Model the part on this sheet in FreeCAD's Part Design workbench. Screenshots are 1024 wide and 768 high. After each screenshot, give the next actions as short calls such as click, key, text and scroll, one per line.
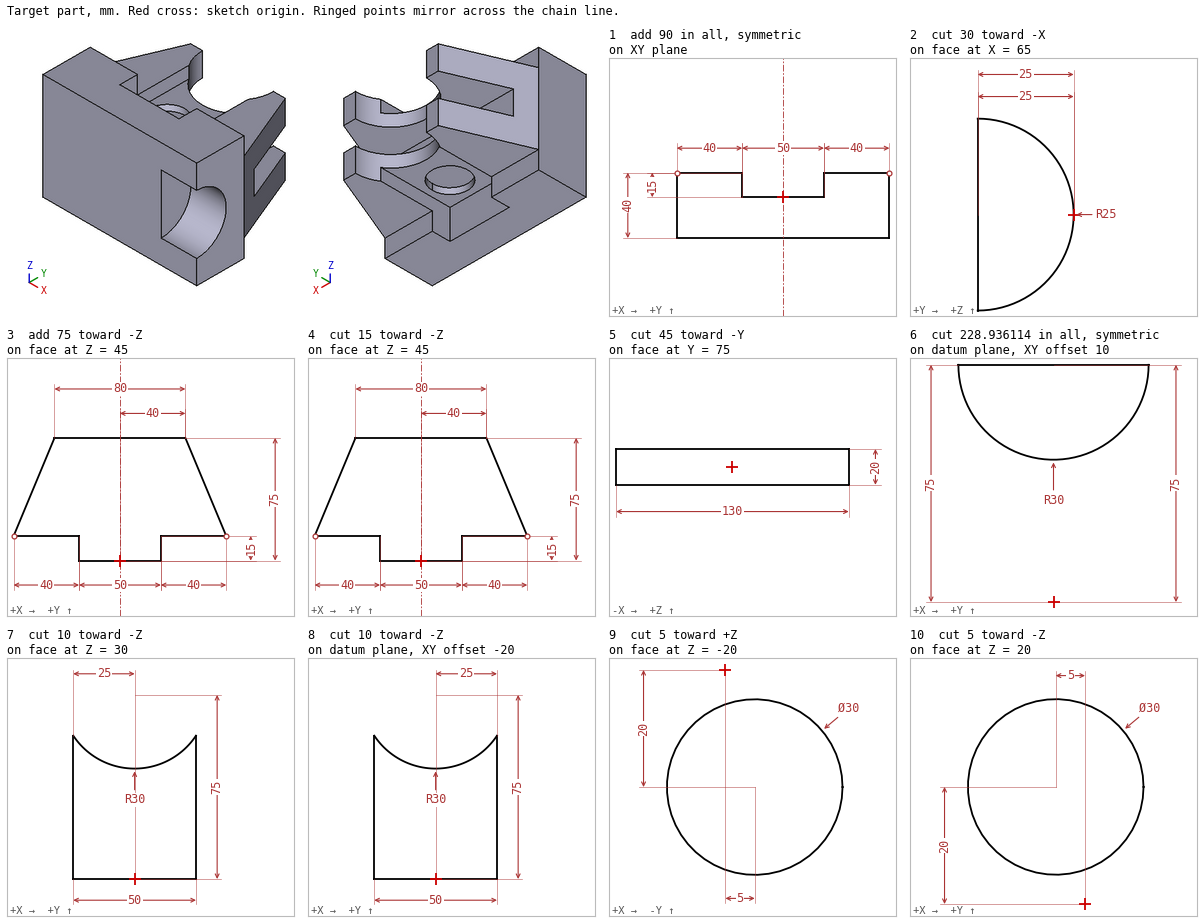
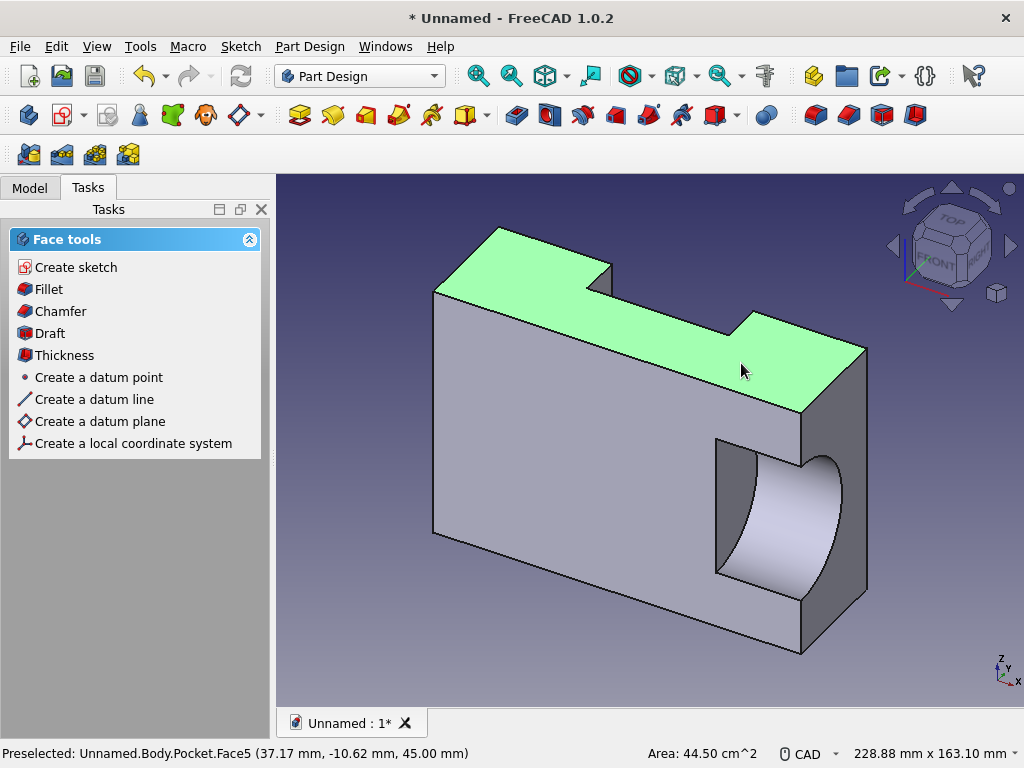
click(62, 116)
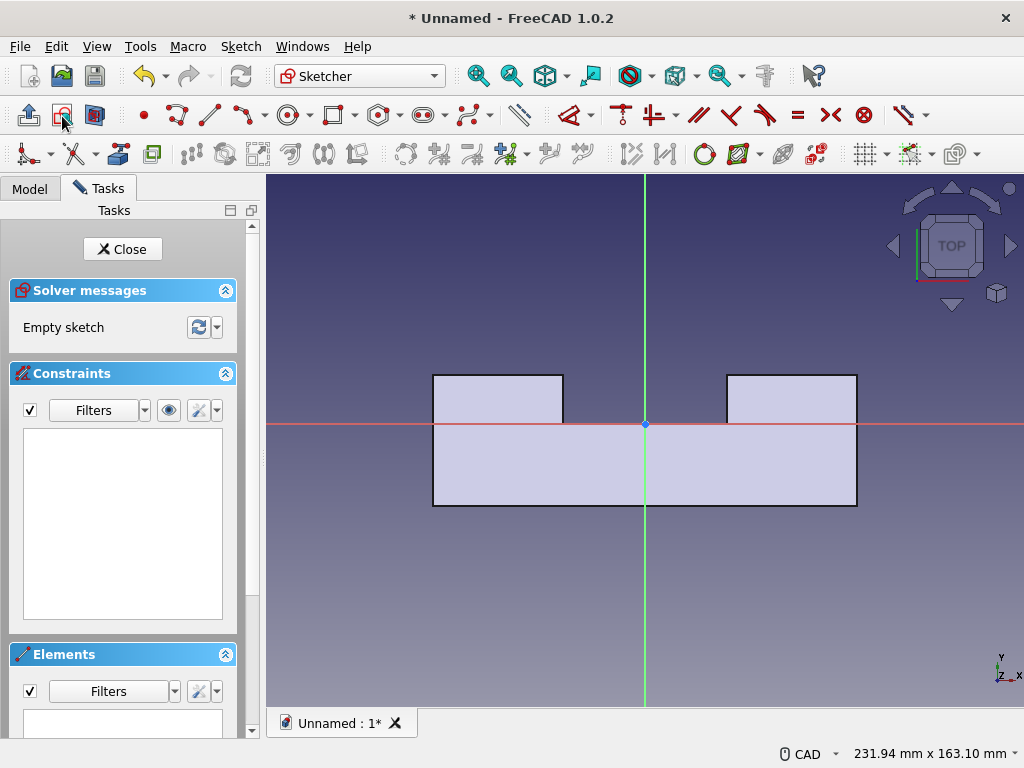
scroll(294, 679, down, 1)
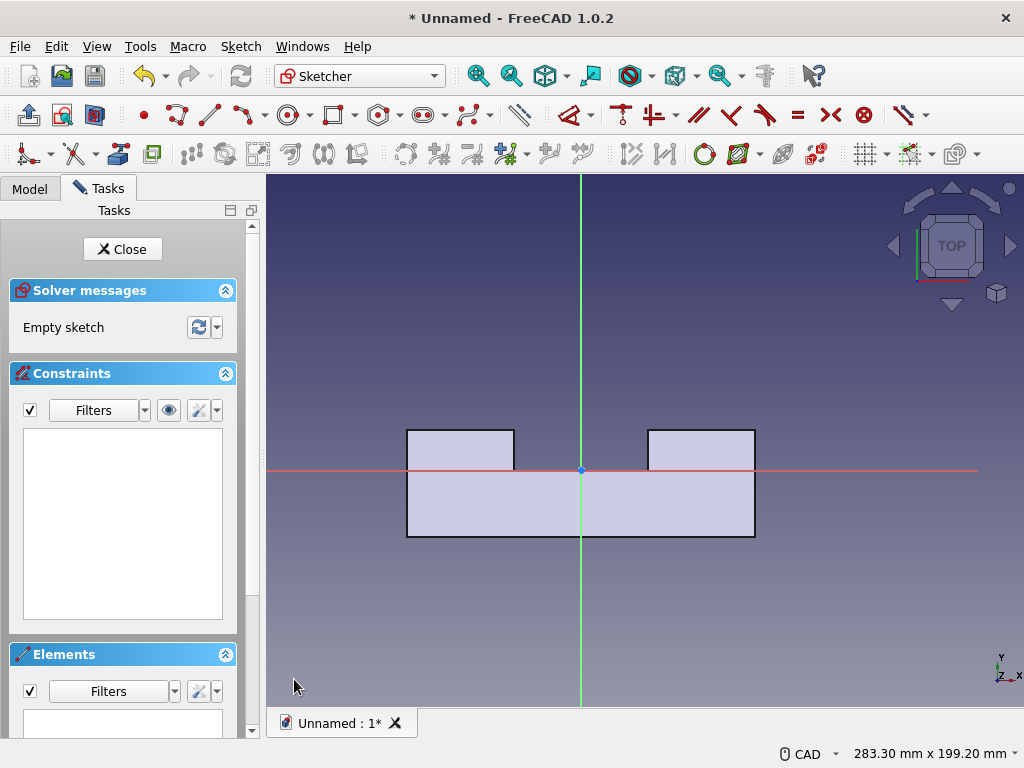
key(g)
key(m)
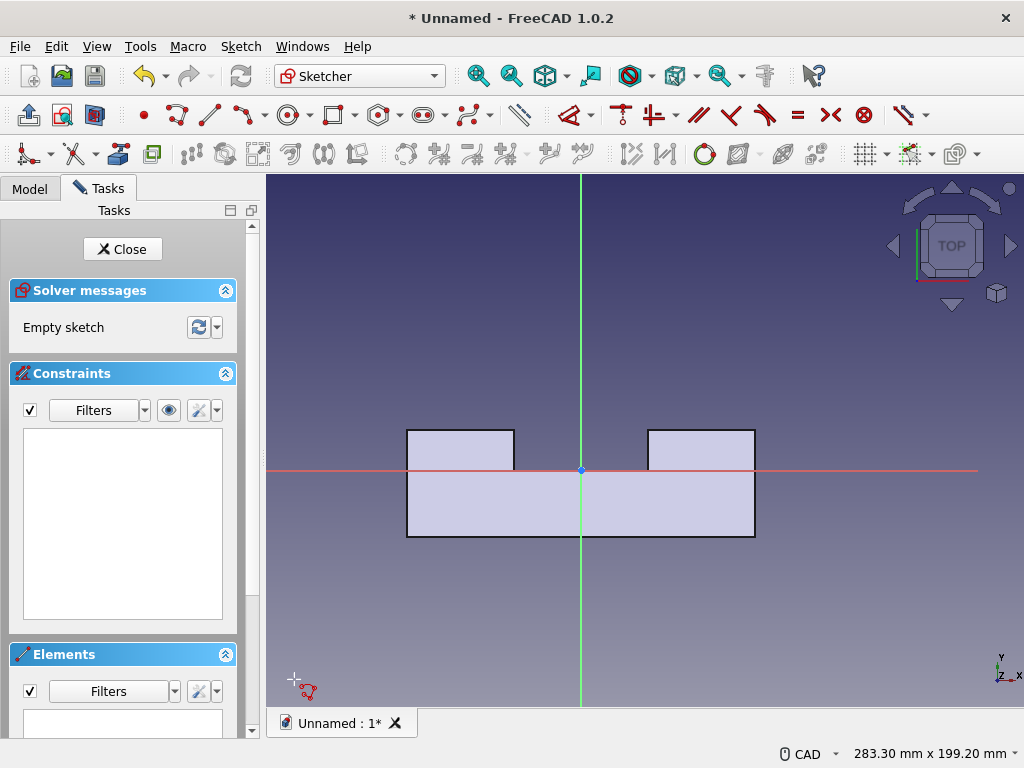
click(514, 471)
click(648, 462)
click(648, 430)
click(755, 430)
click(688, 270)
click(474, 270)
click(407, 430)
click(514, 430)
click(514, 471)
key(Escape)
key(Escape)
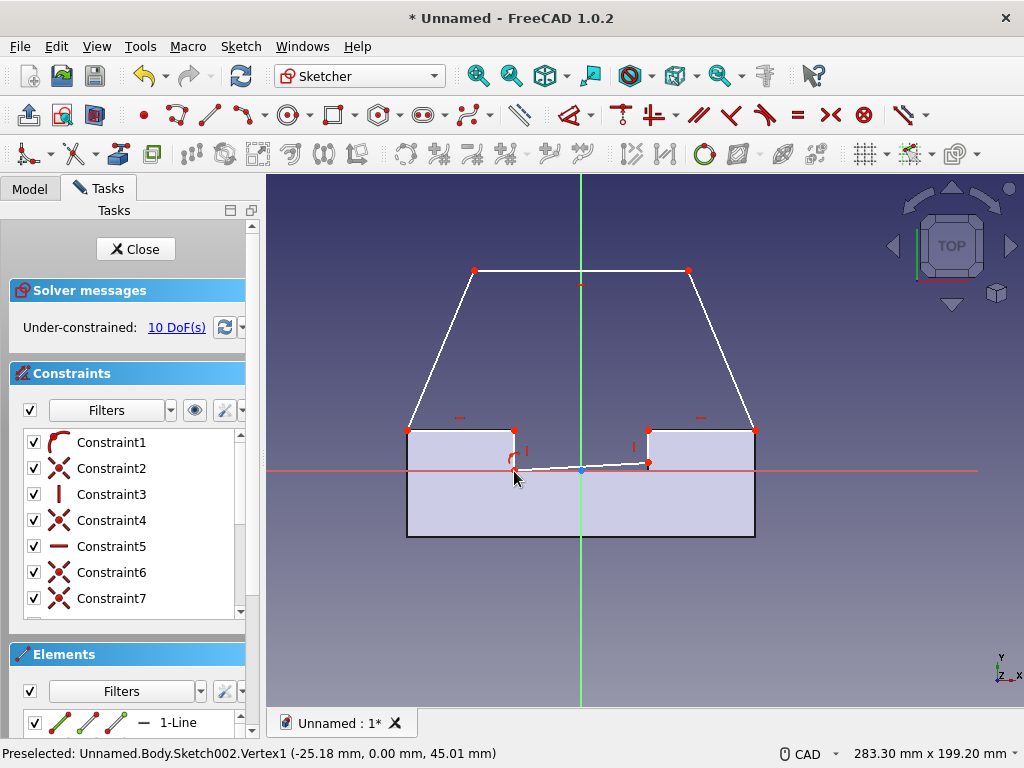
click(554, 468)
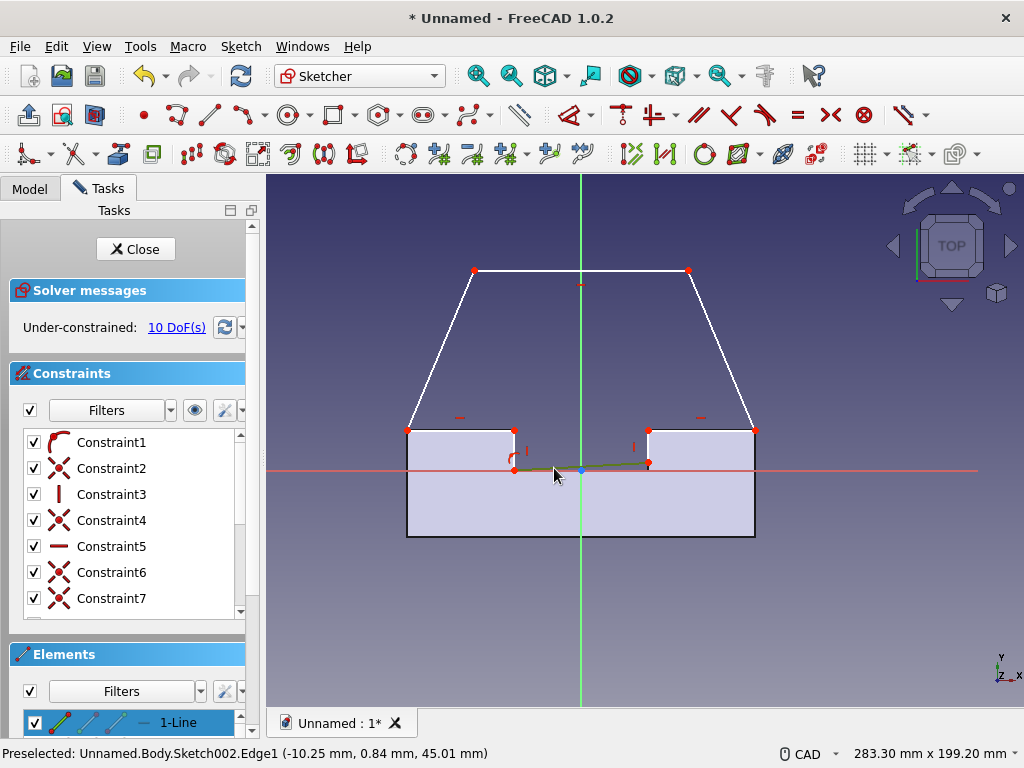
key(h)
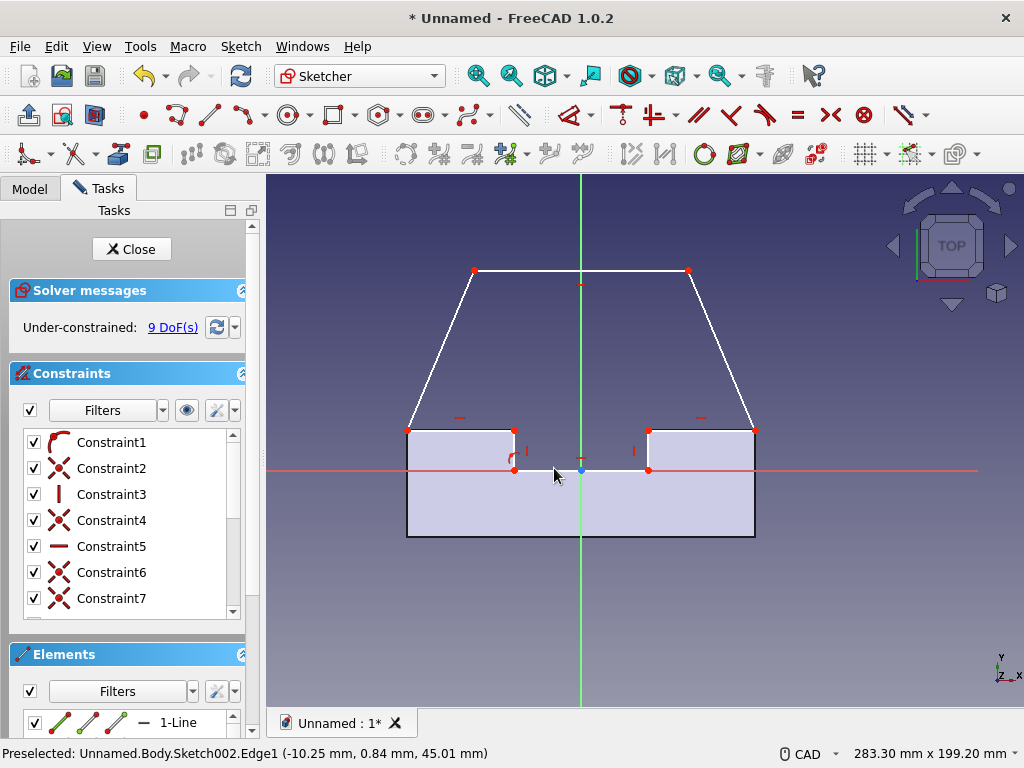
click(755, 431)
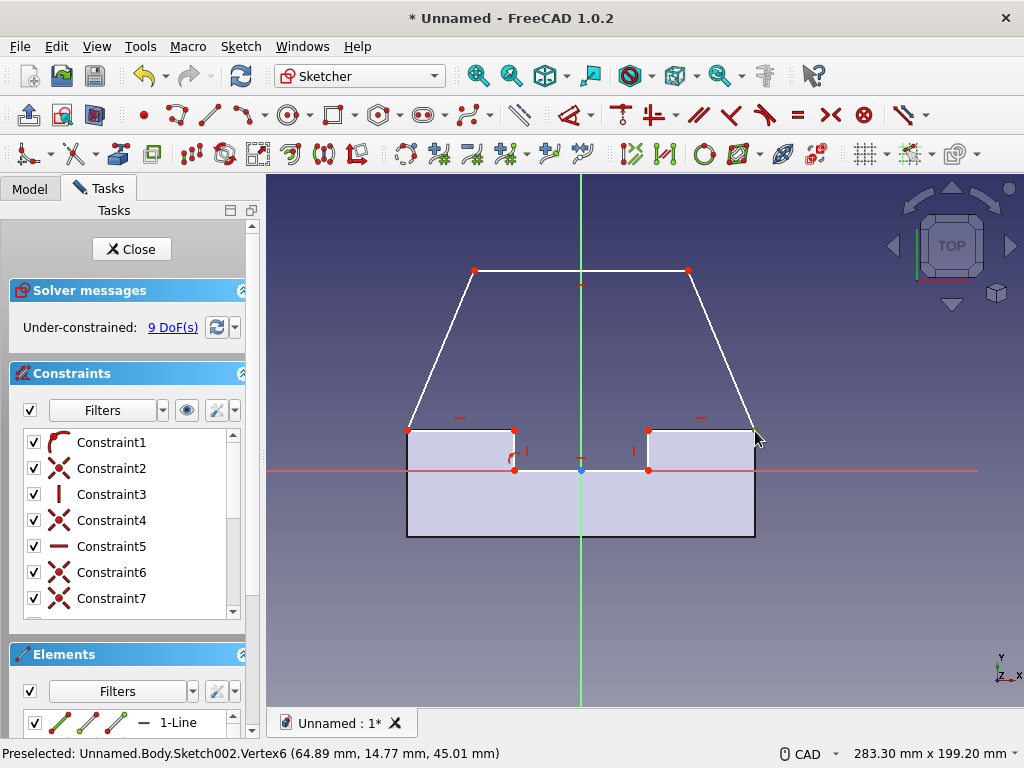
click(407, 431)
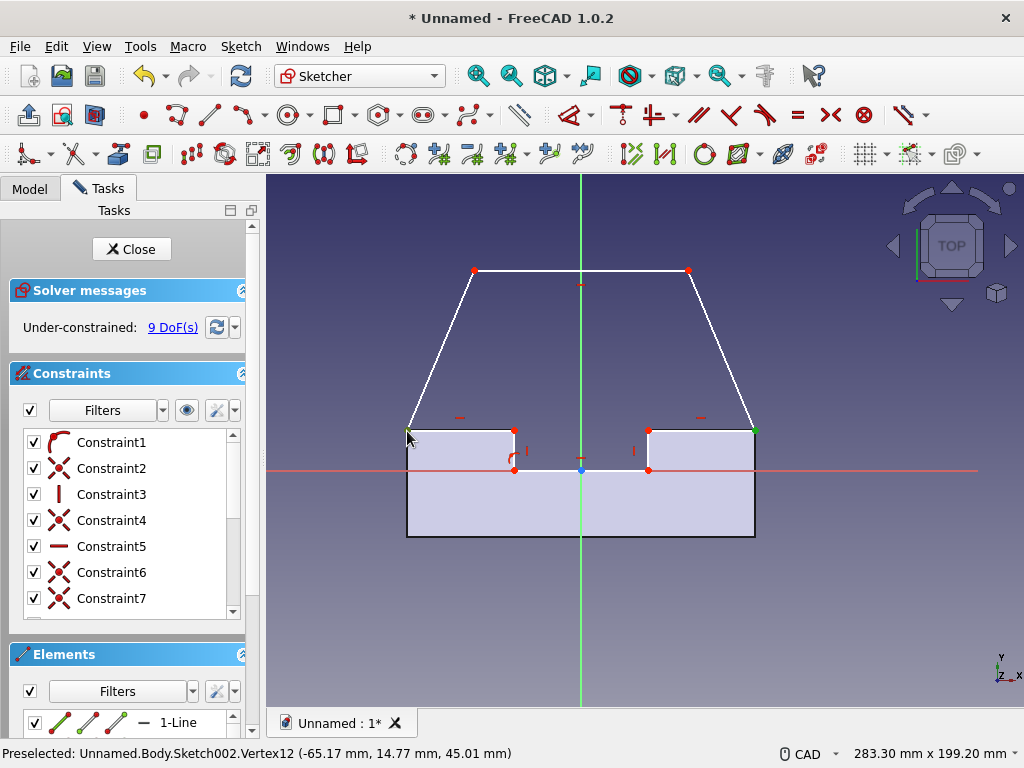
click(581, 645)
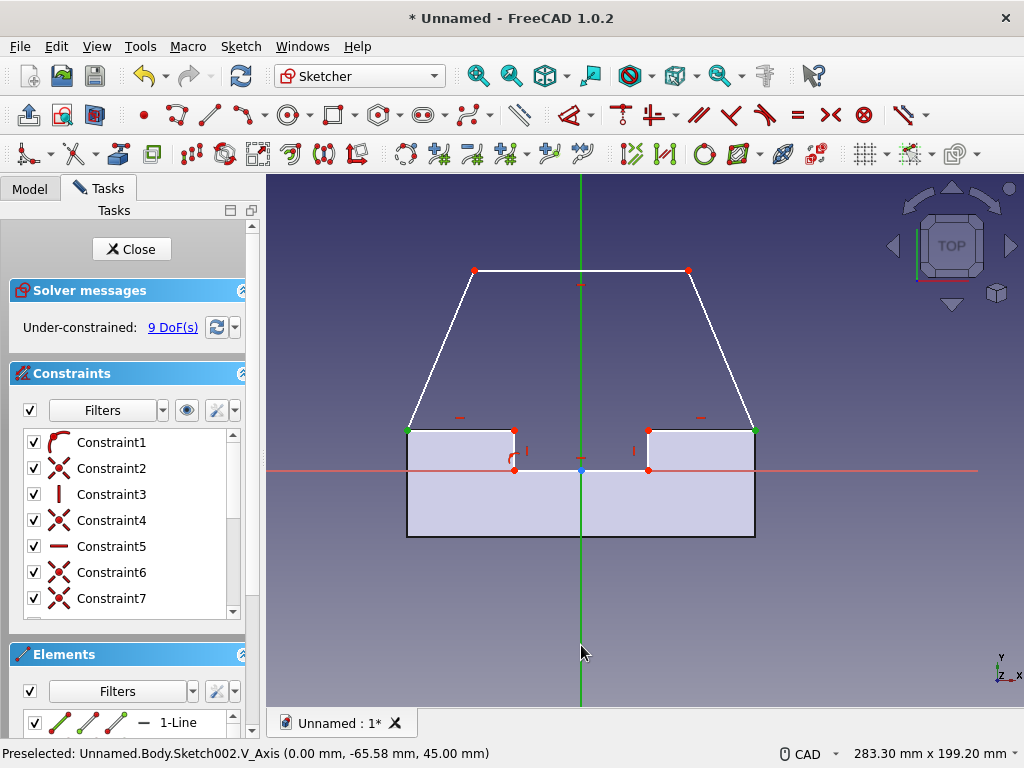
key(s)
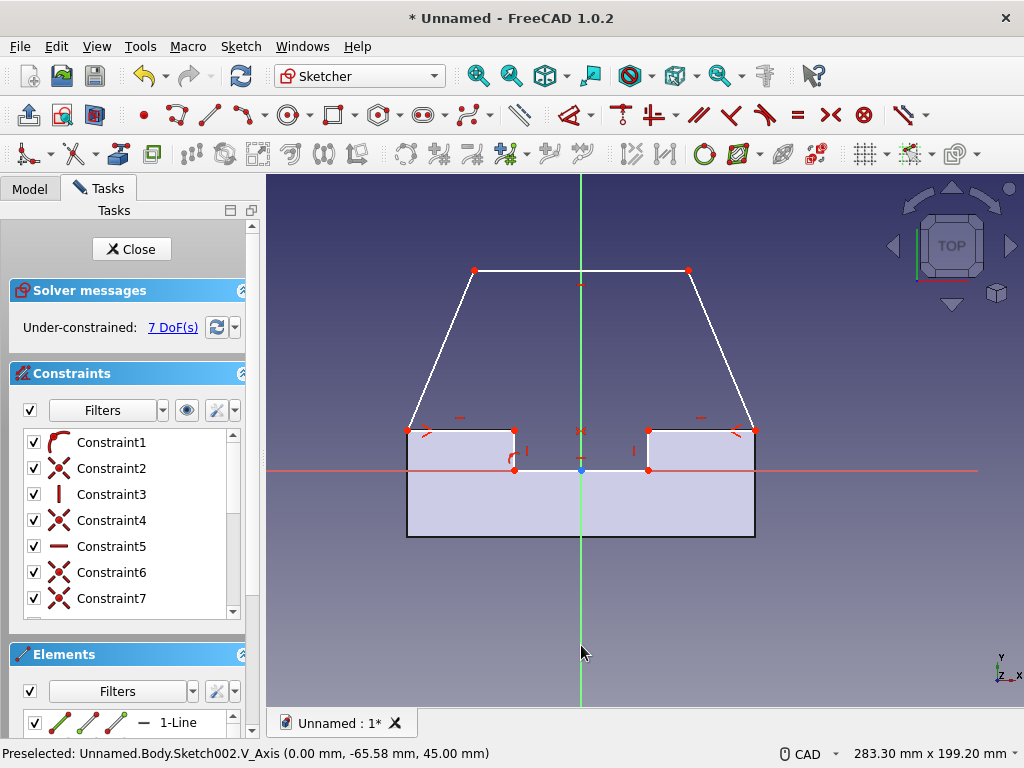
click(568, 116)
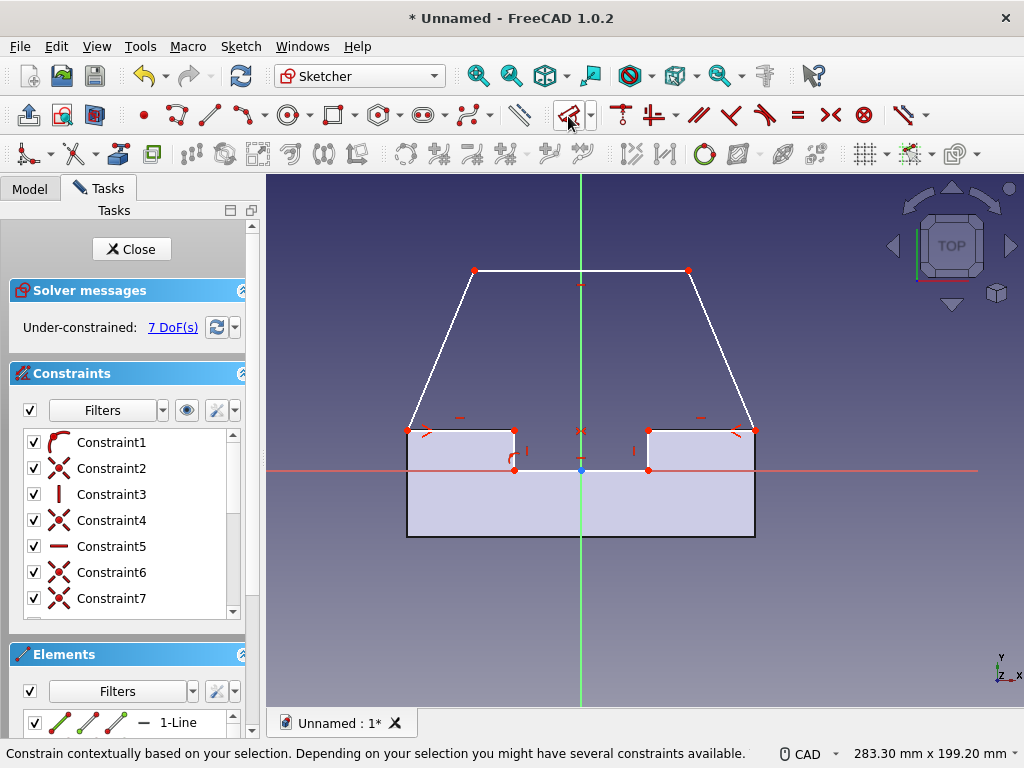
click(554, 471)
click(550, 505)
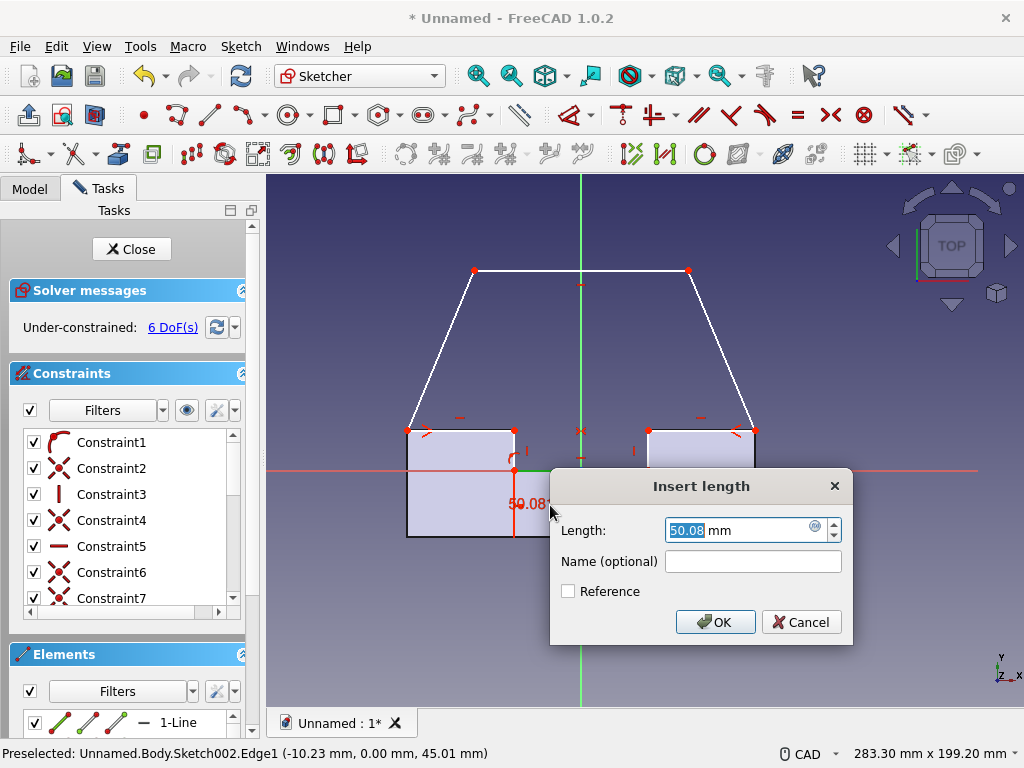
text(50)
key(Return)